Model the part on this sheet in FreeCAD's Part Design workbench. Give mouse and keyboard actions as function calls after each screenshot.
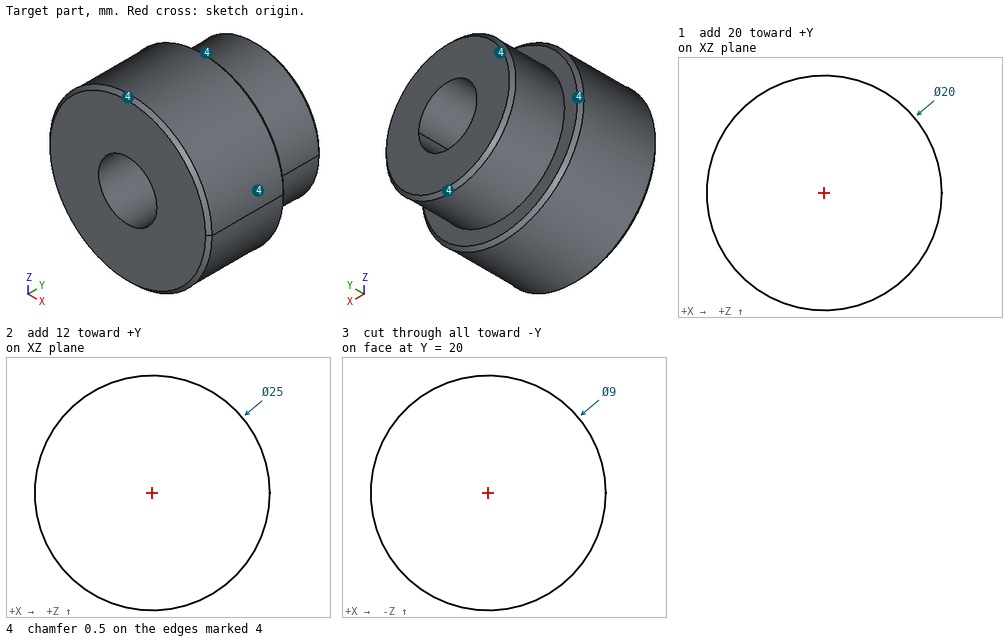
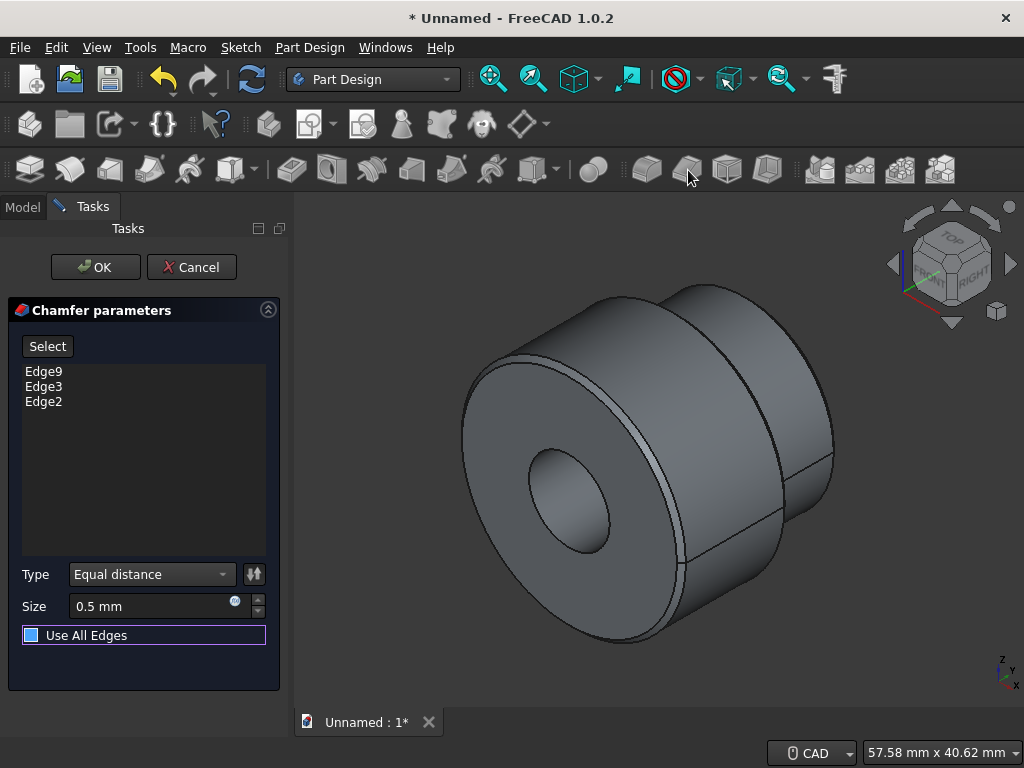
click(96, 267)